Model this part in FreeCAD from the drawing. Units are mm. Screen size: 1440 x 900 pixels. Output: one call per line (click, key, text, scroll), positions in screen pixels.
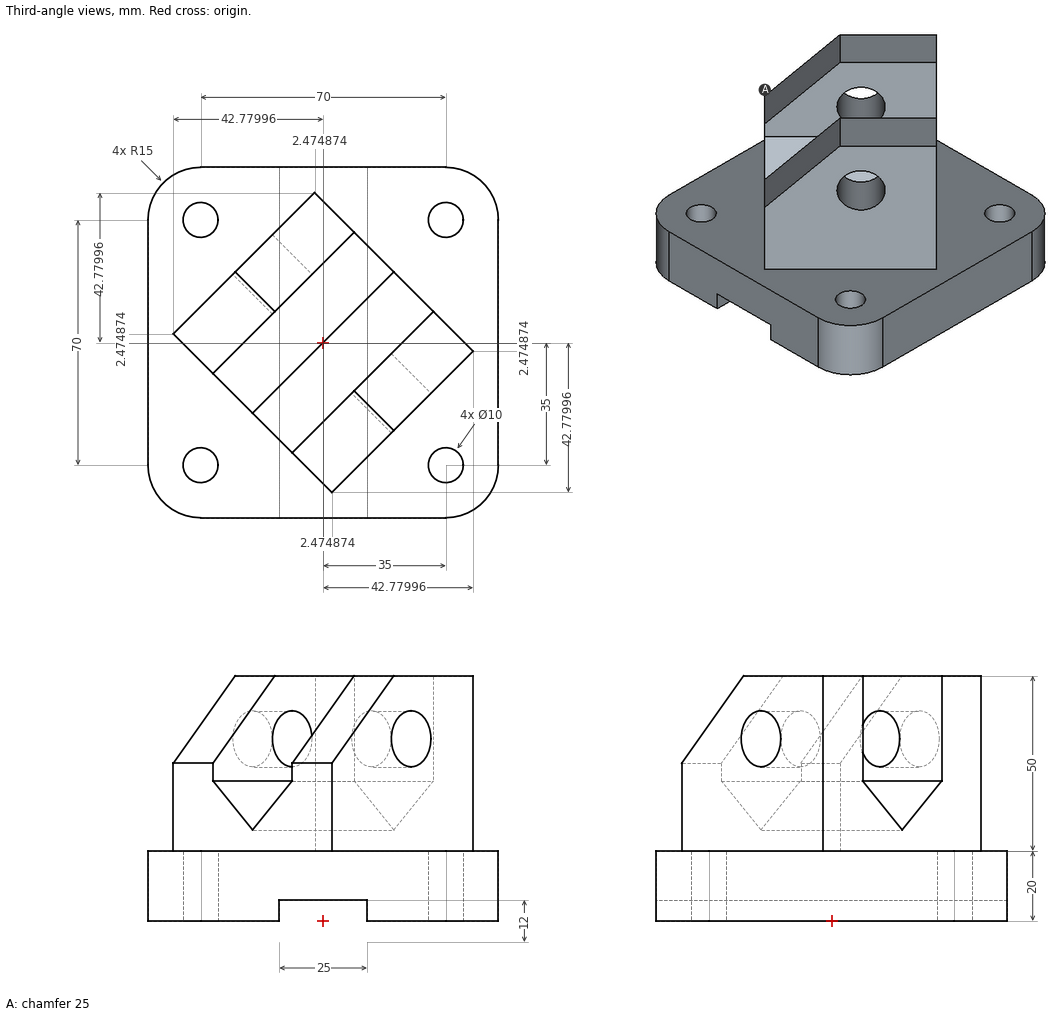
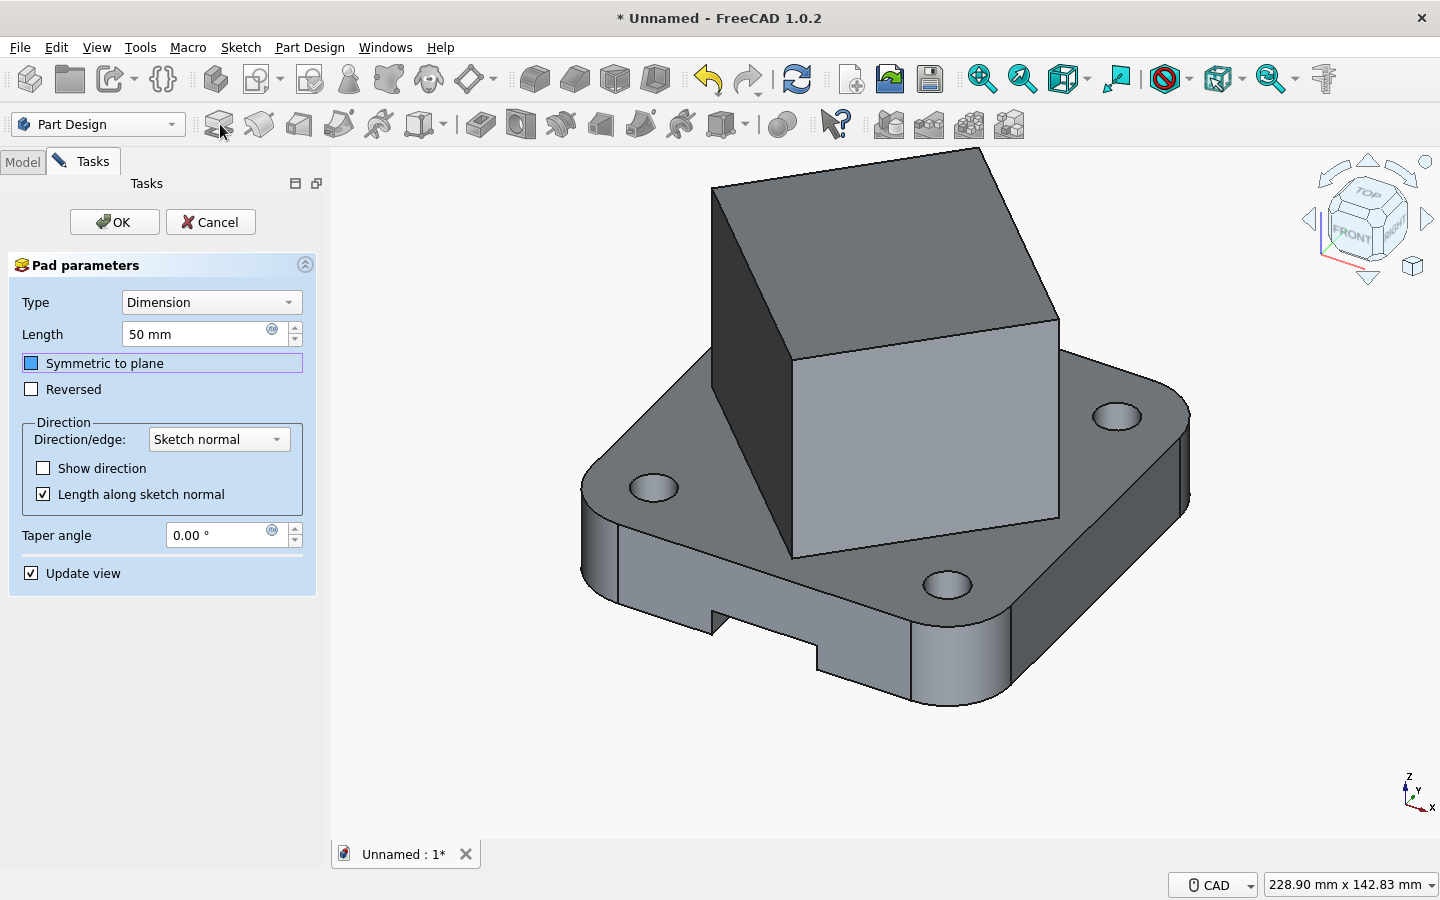
click(115, 222)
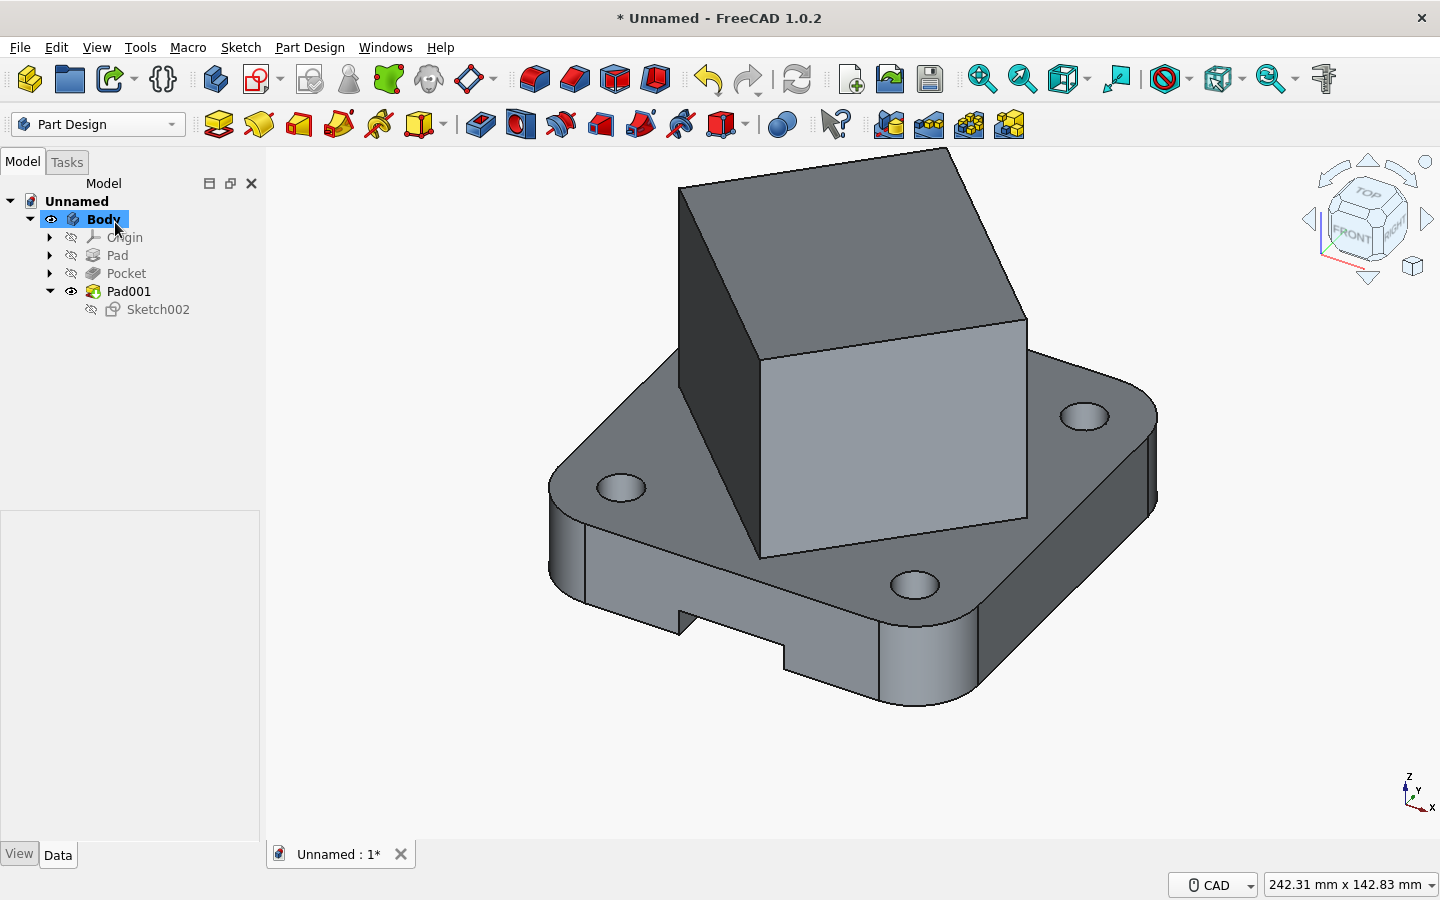
key(v)
key(f)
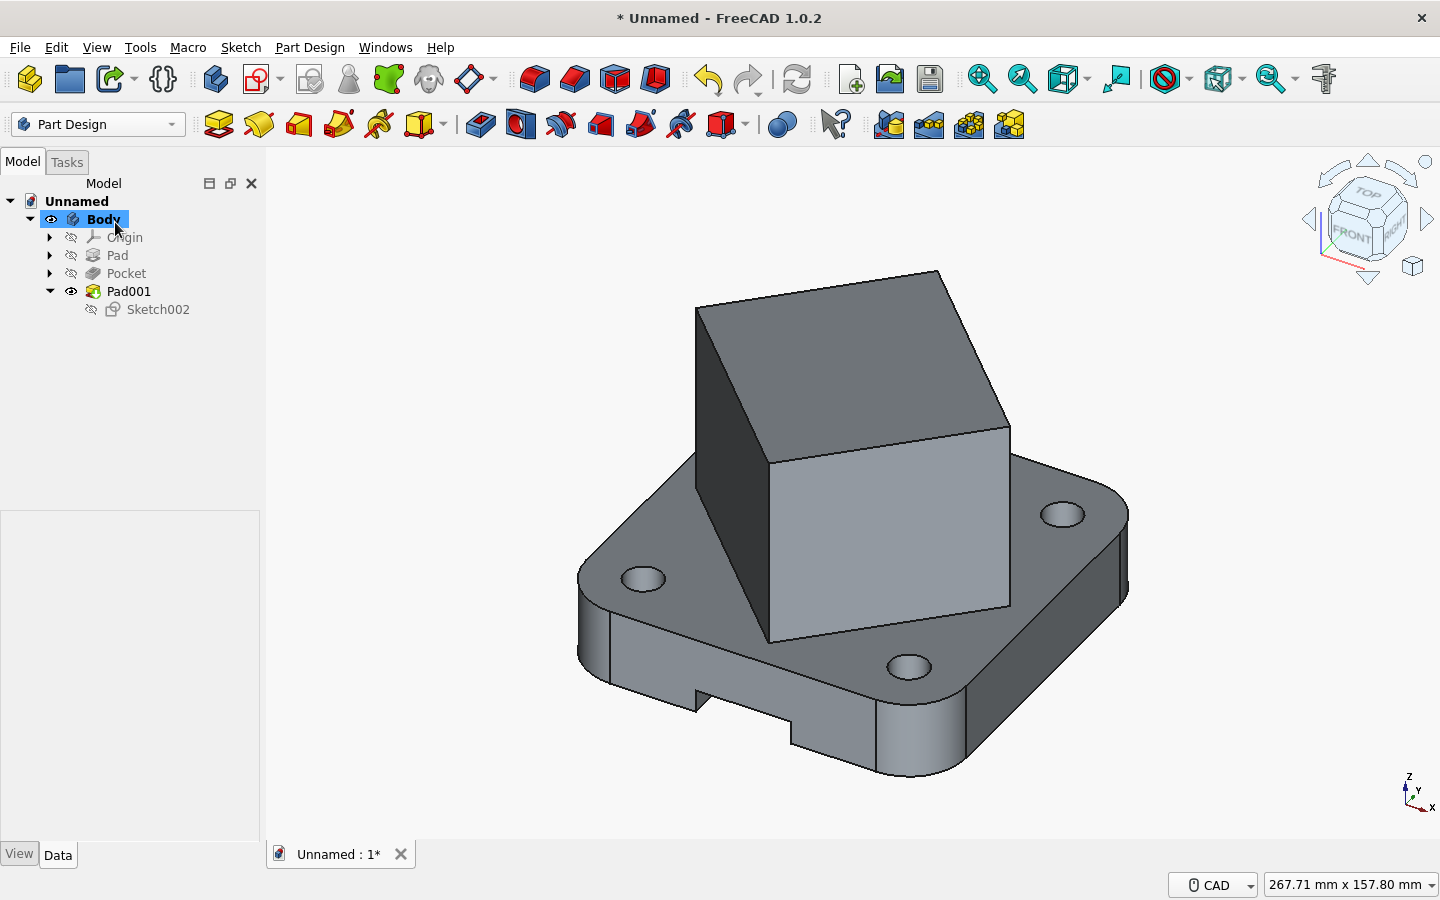
click(889, 534)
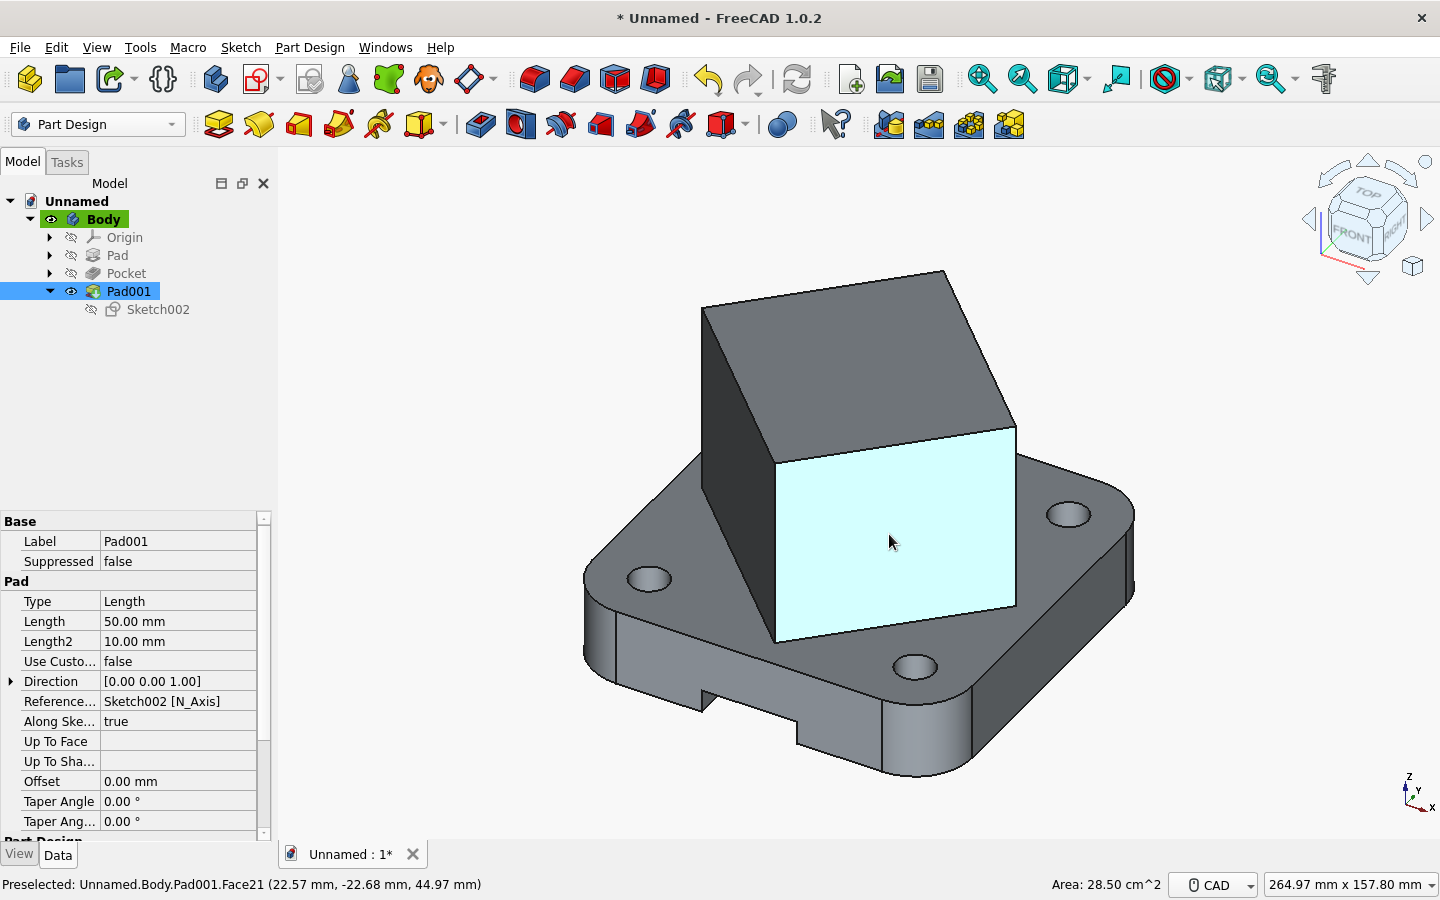
click(256, 80)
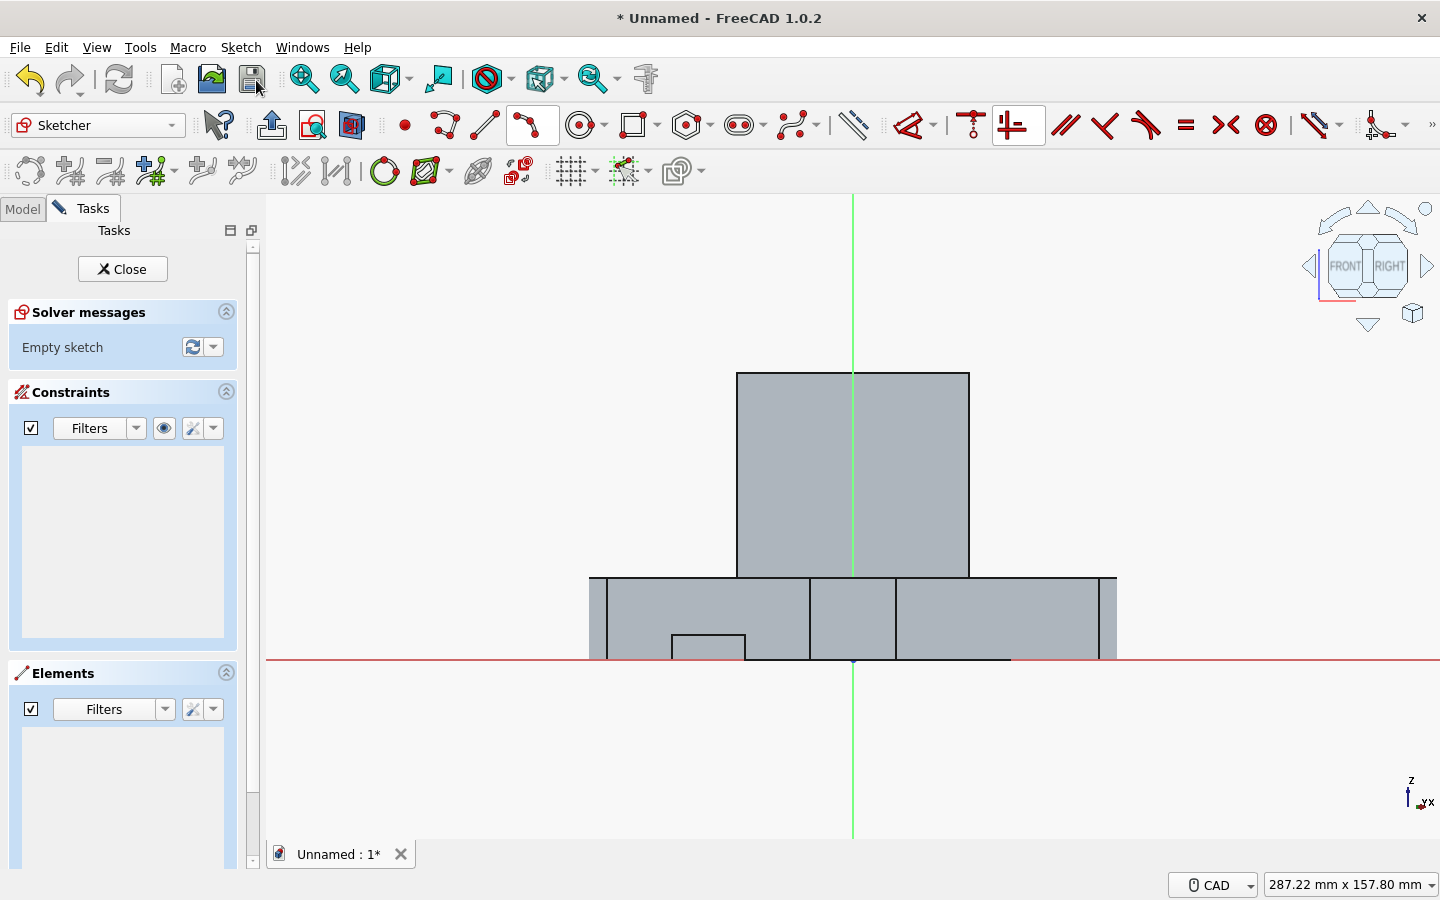
key(q)
key(s)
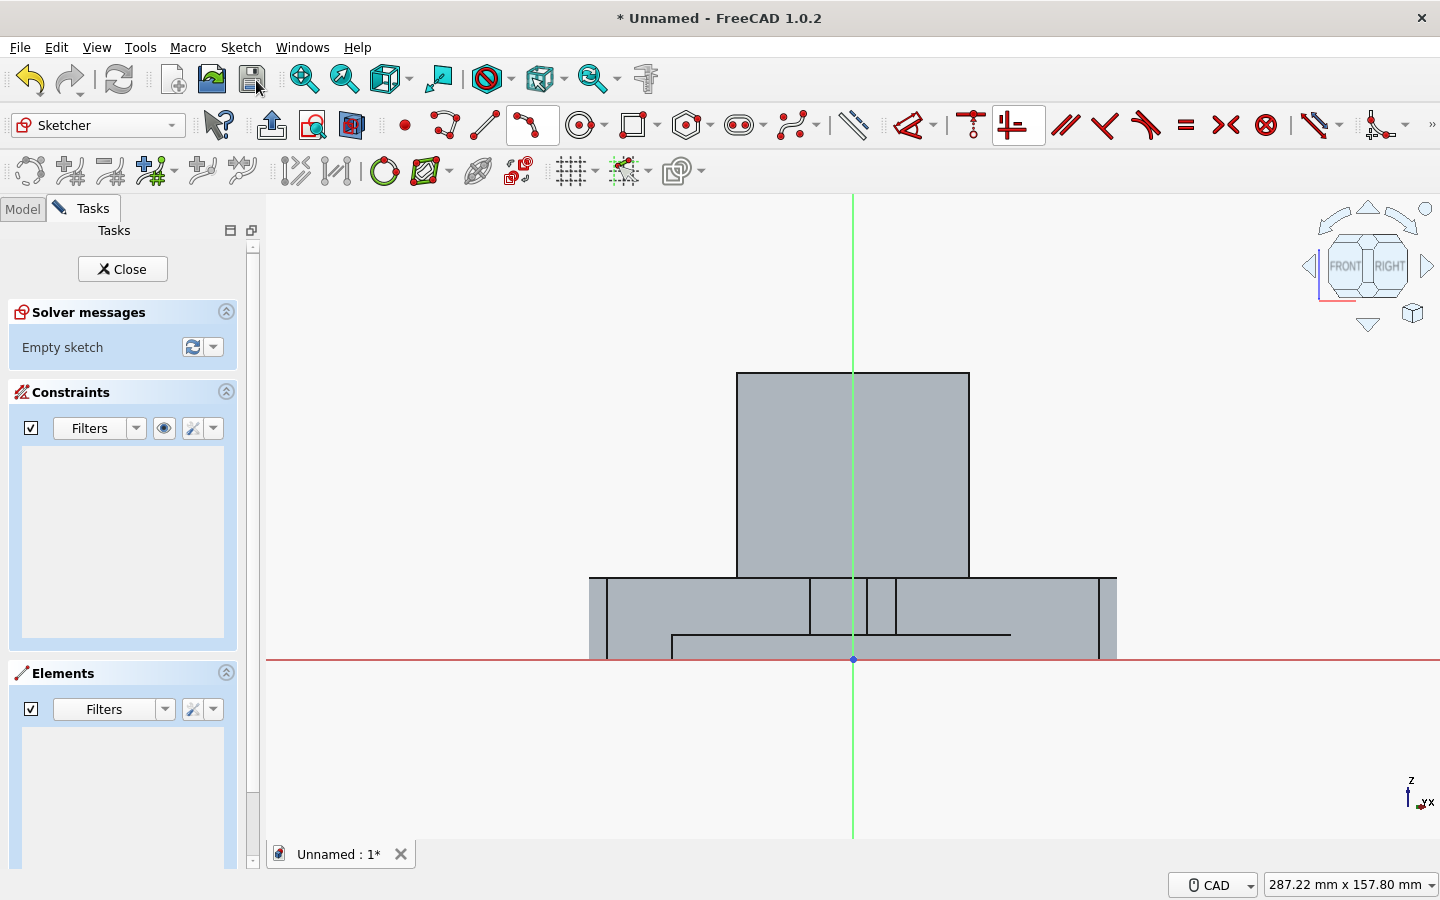
scroll(884, 433, up, 9)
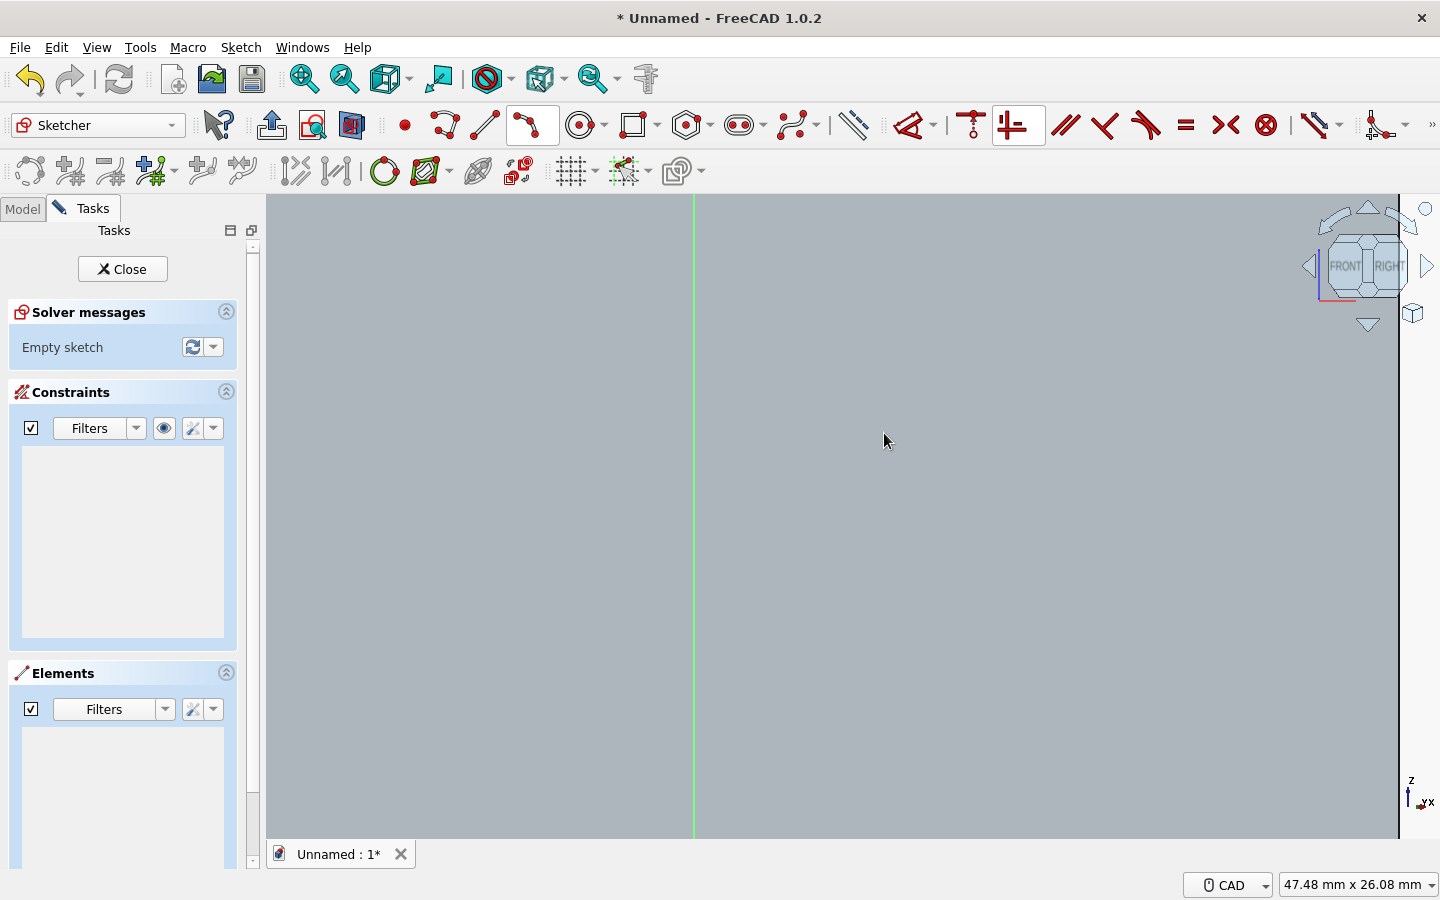
key(g)
key(c)